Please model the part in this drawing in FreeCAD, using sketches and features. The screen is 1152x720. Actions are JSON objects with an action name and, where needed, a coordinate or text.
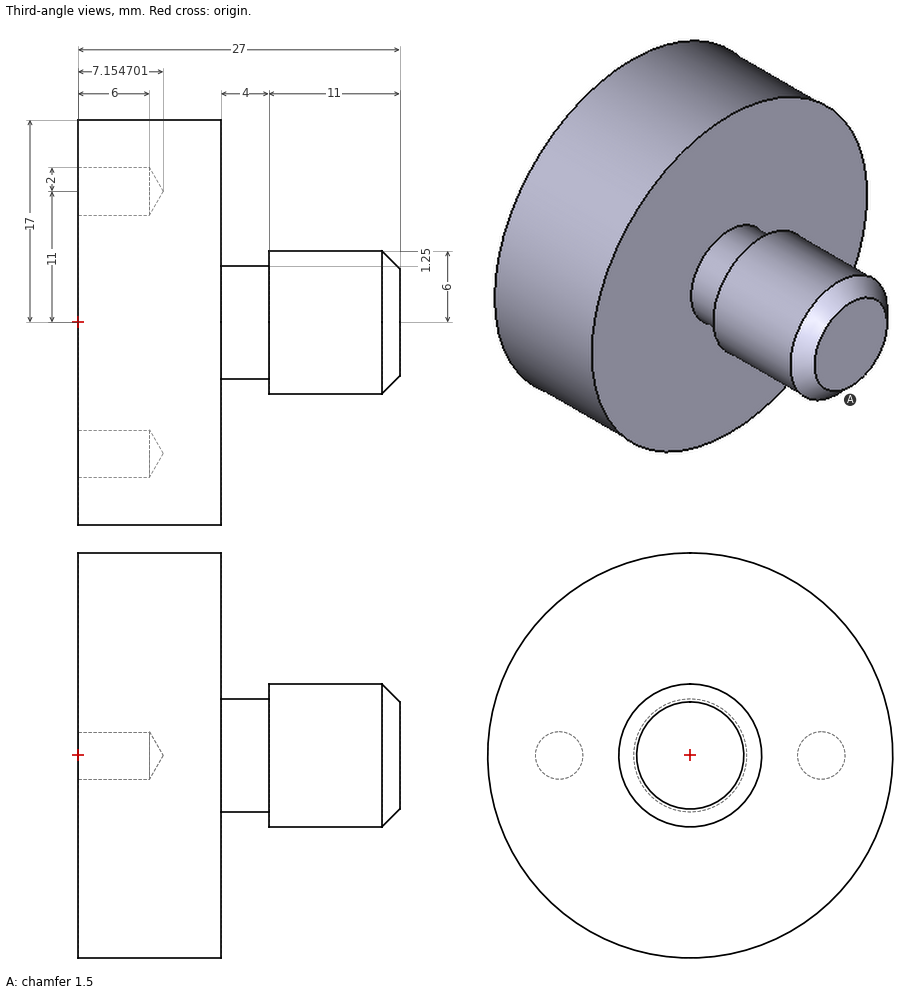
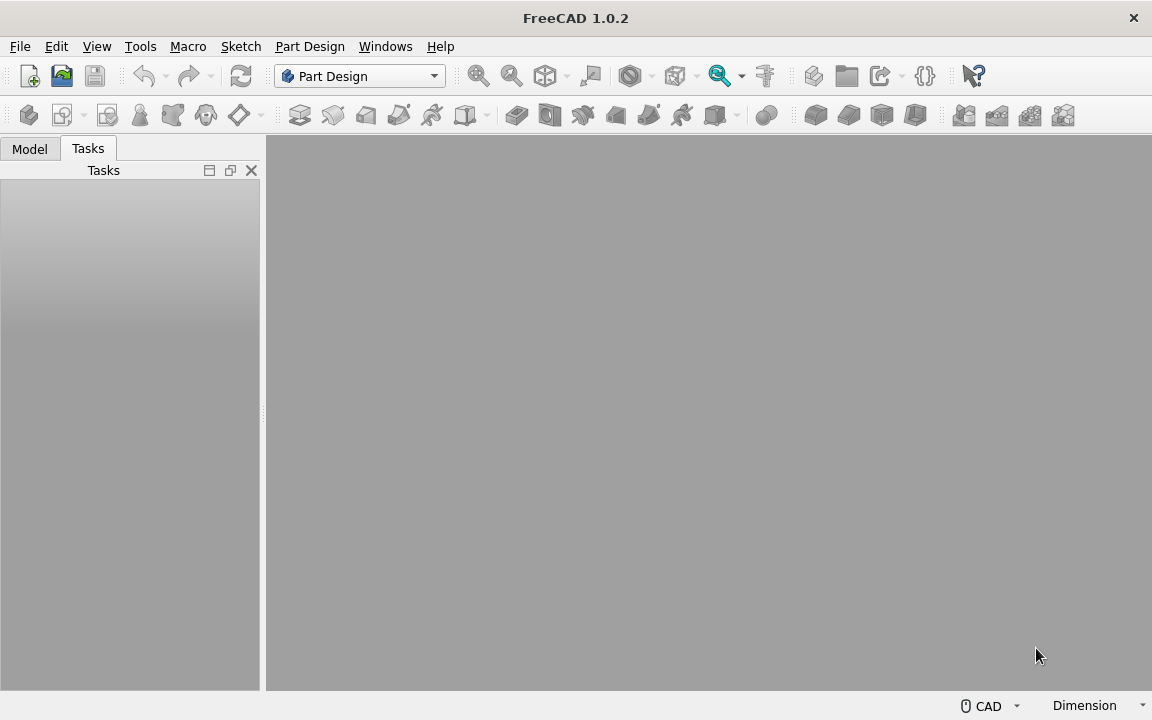
{"action": "left_click", "coordinate": [29, 76]}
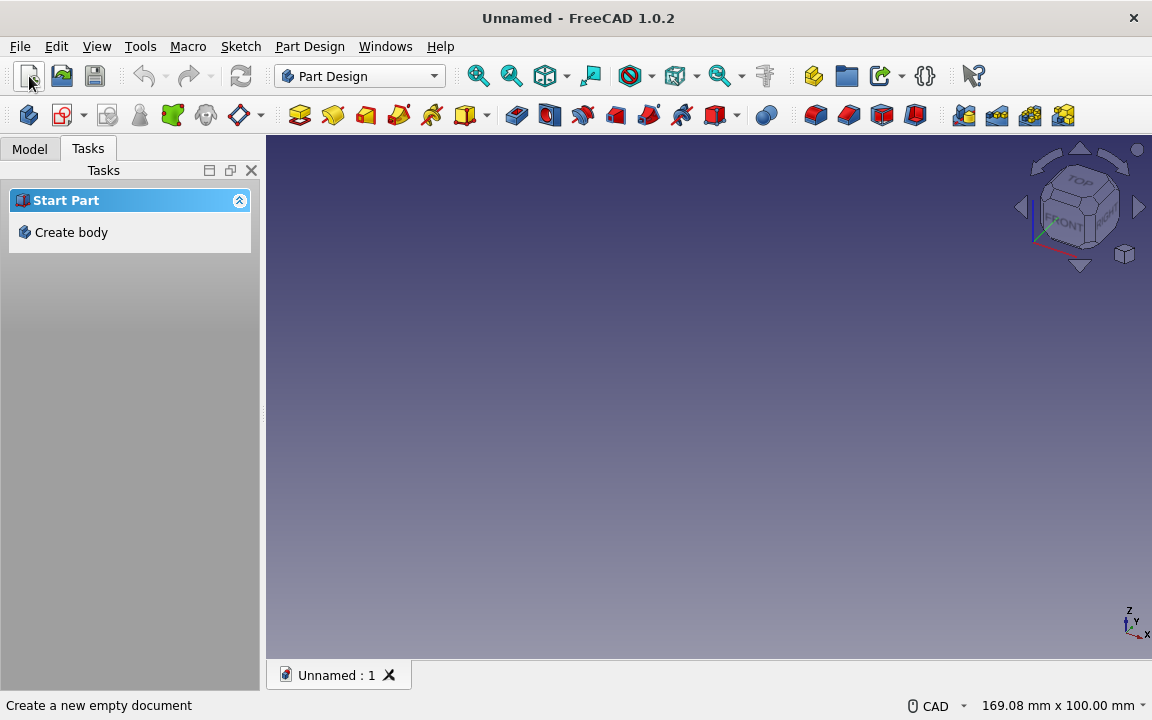
{"action": "left_click", "coordinate": [62, 116]}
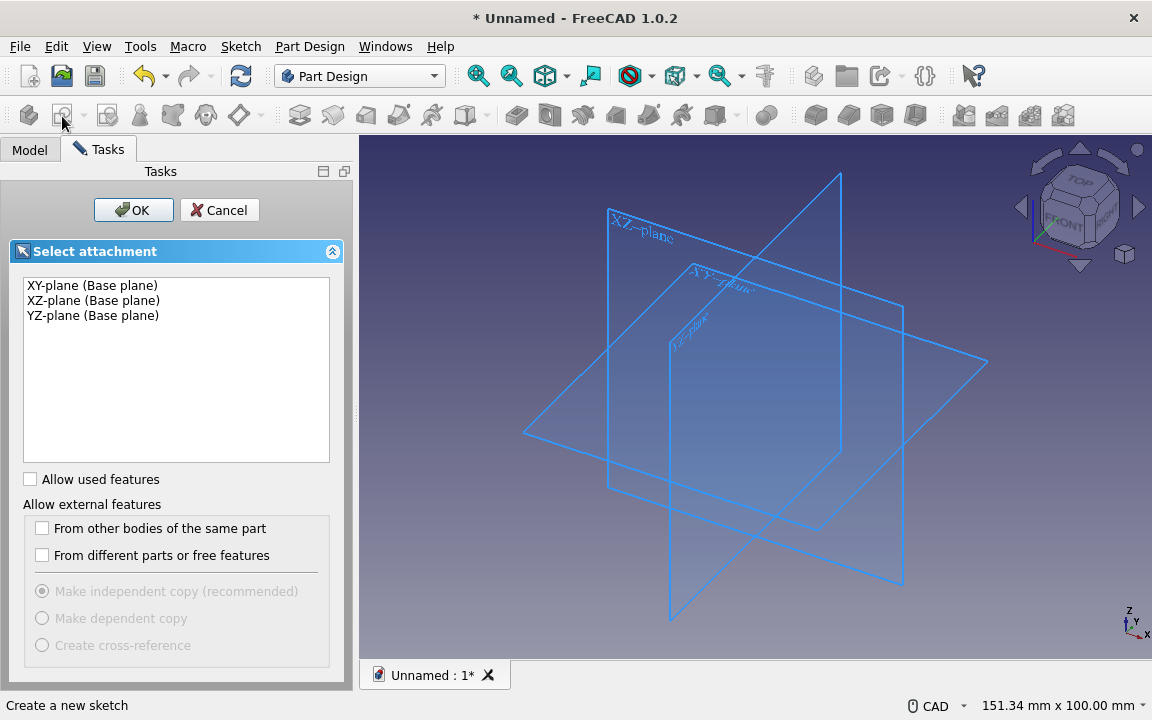
{"action": "left_click", "coordinate": [84, 286]}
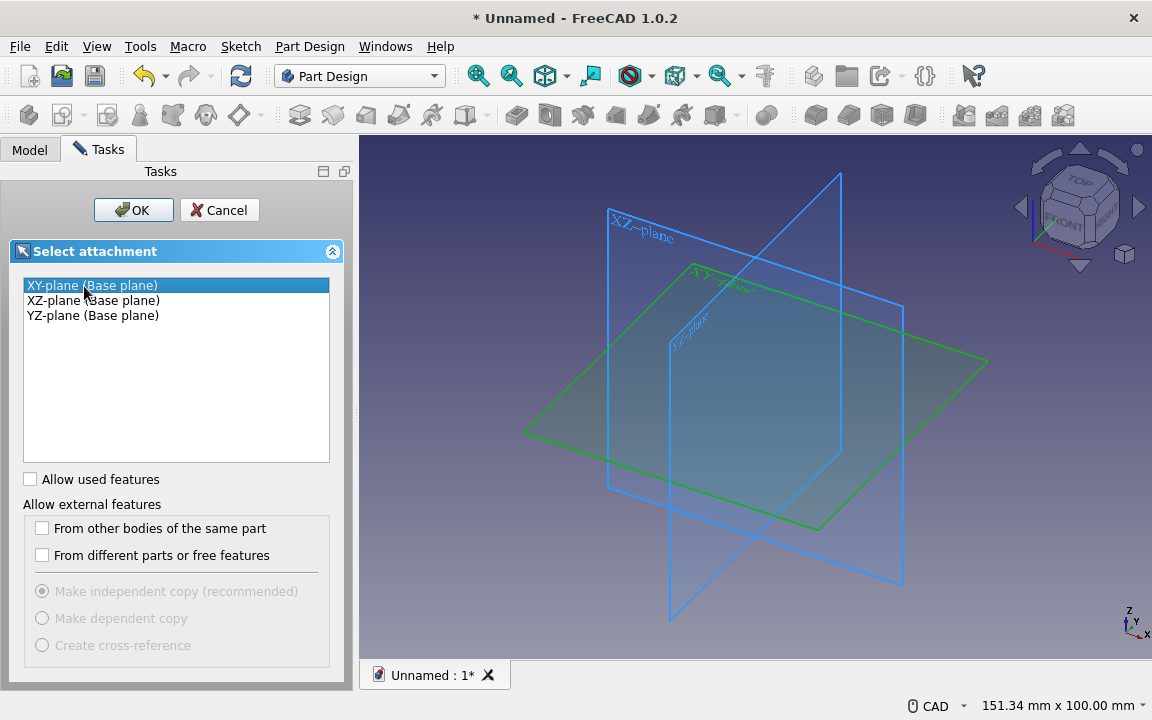
{"action": "left_click", "coordinate": [134, 210]}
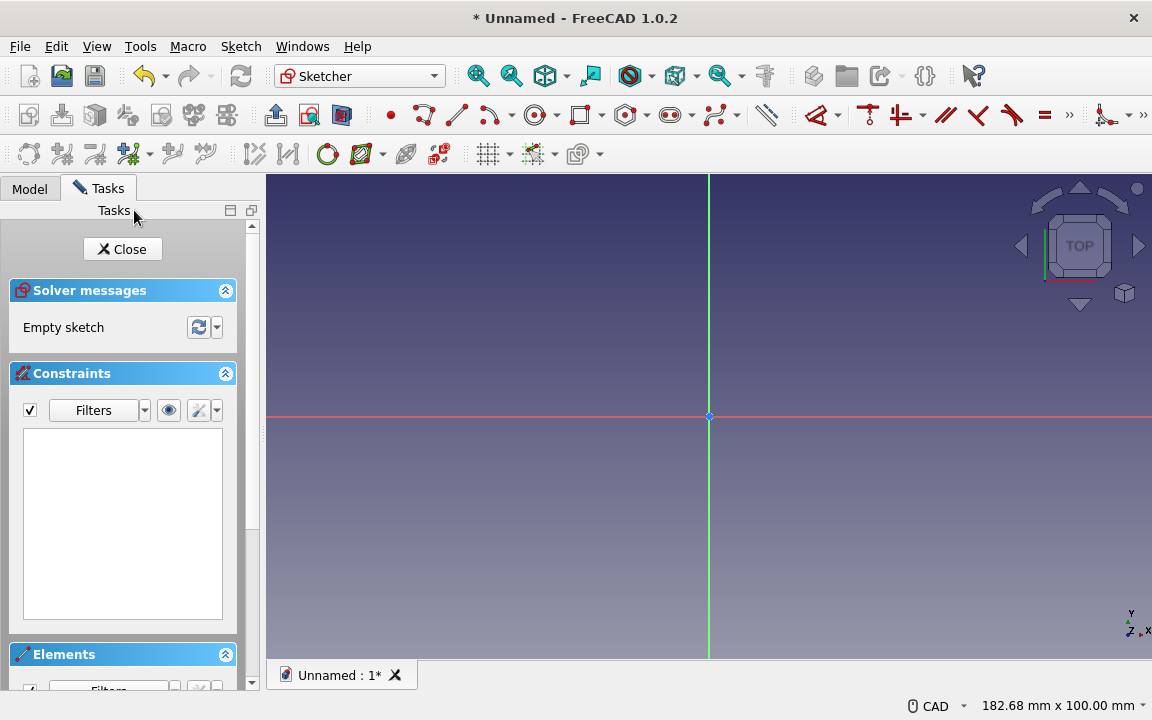
{"action": "scroll", "coordinate": [818, 362], "scroll_direction": "up", "scroll_amount": 7}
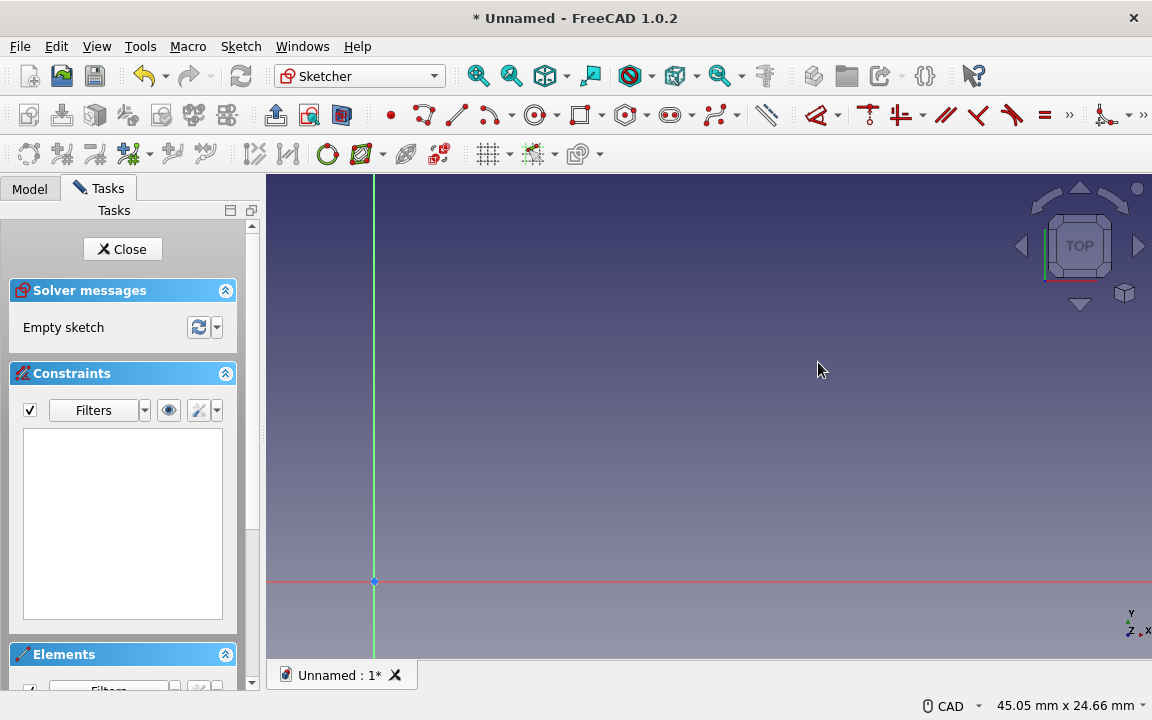
{"action": "key", "text": "g m"}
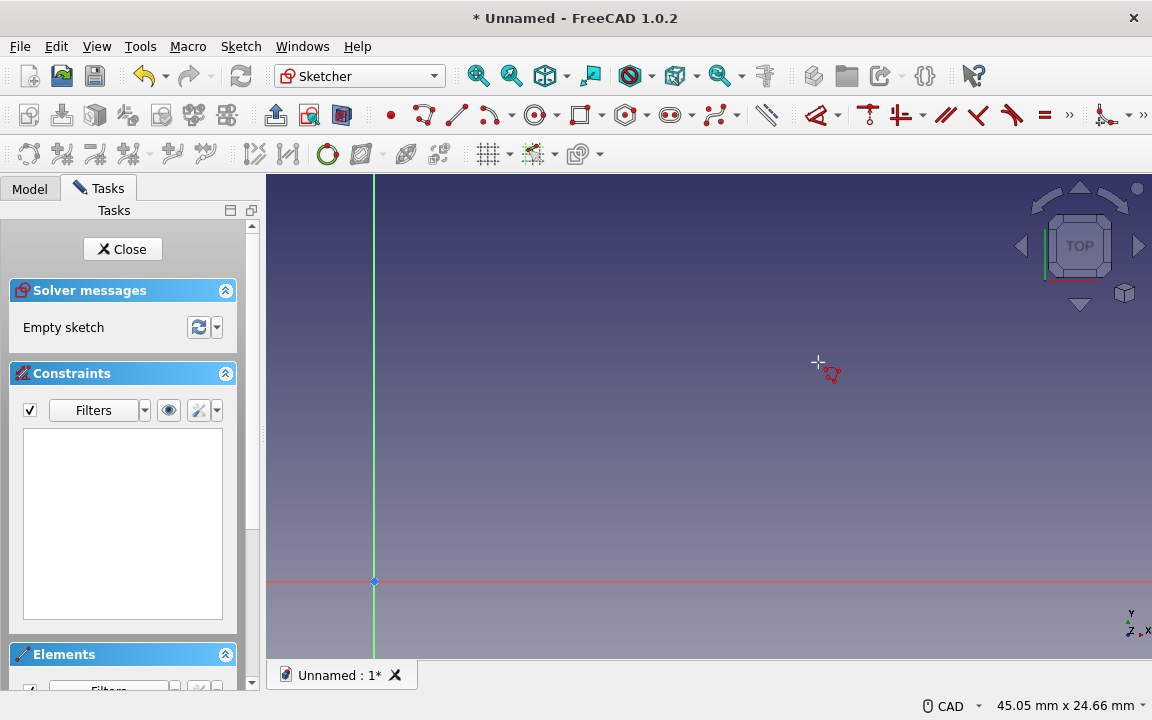
{"action": "left_click", "coordinate": [374, 582]}
{"action": "left_click", "coordinate": [905, 573]}
{"action": "left_click", "coordinate": [905, 464]}
{"action": "left_click", "coordinate": [689, 464]}
{"action": "left_click", "coordinate": [689, 488]}
{"action": "left_click", "coordinate": [610, 488]}
{"action": "left_click", "coordinate": [610, 247]}
{"action": "left_click", "coordinate": [383, 247]}
{"action": "left_click", "coordinate": [374, 582]}
{"action": "key", "text": "Escape"}
{"action": "key", "text": "Escape"}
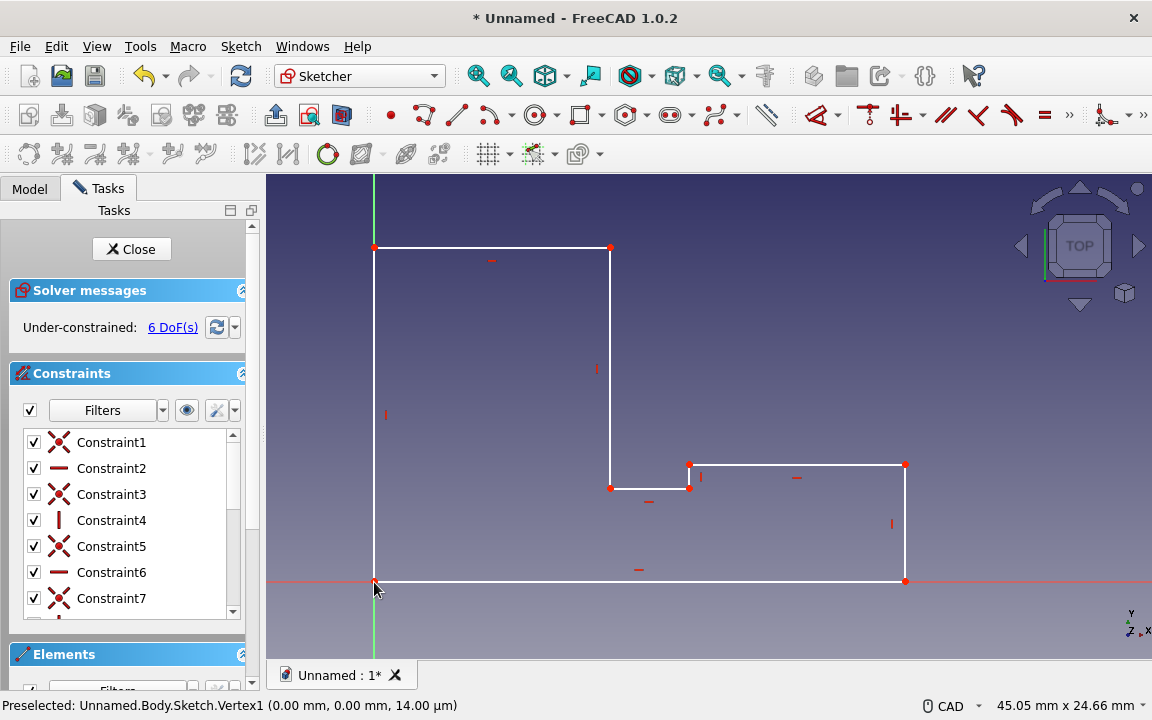
{"action": "left_click", "coordinate": [816, 116]}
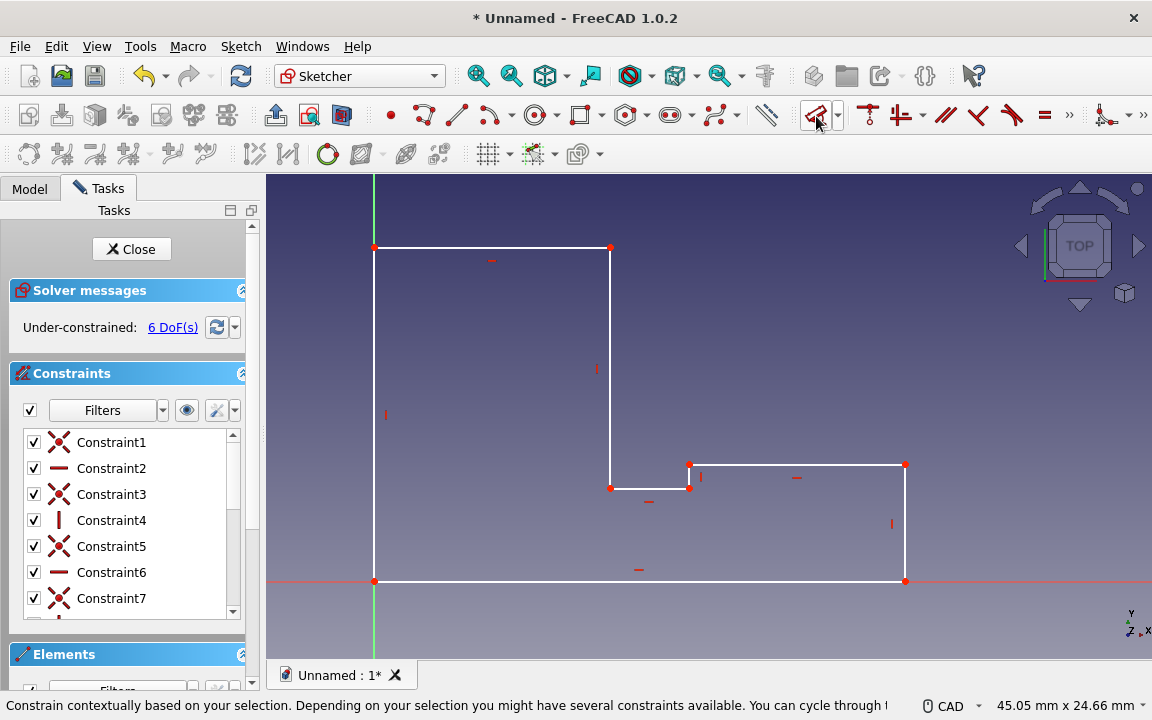
{"action": "left_click", "coordinate": [905, 547]}
{"action": "left_click", "coordinate": [939, 523]}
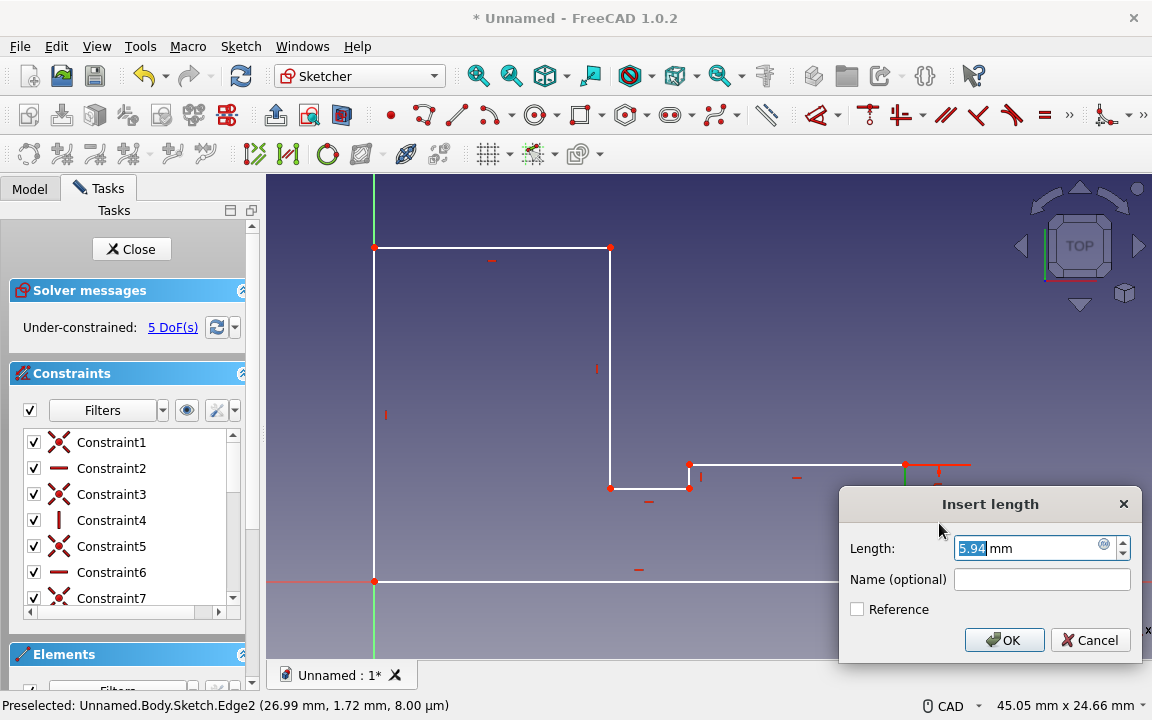
{"action": "type", "text": "6"}
{"action": "key", "text": "Return"}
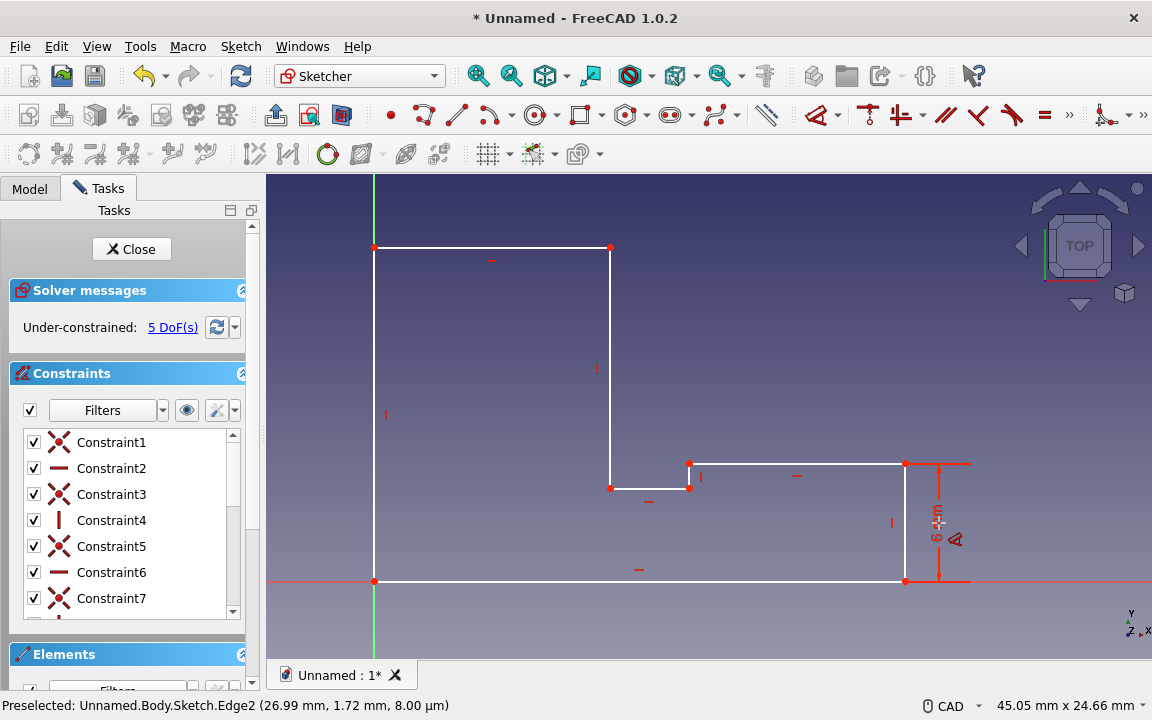
{"action": "left_click", "coordinate": [665, 489]}
{"action": "left_click", "coordinate": [650, 523]}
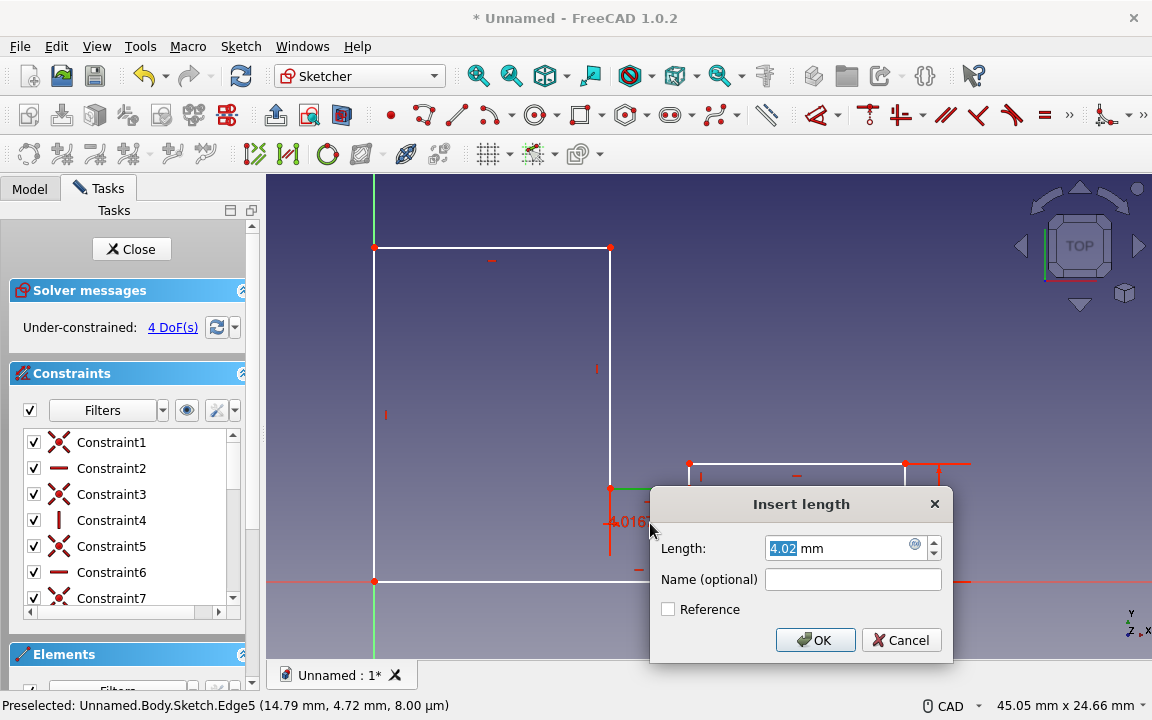
{"action": "type", "text": "4"}
{"action": "key", "text": "Return"}